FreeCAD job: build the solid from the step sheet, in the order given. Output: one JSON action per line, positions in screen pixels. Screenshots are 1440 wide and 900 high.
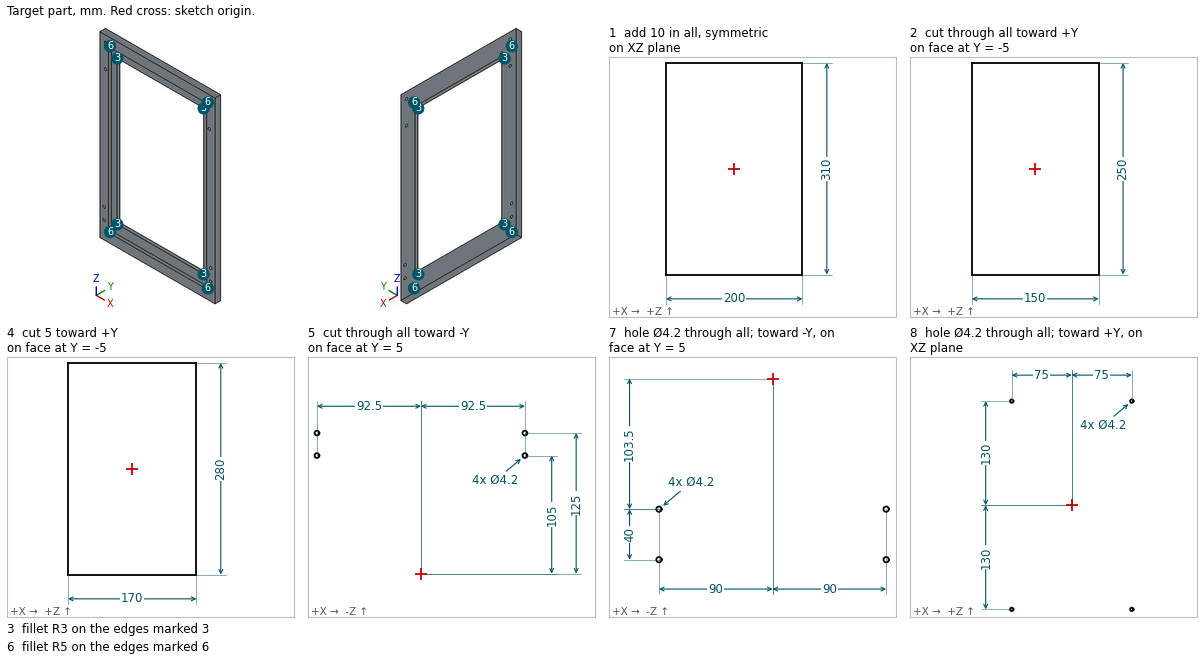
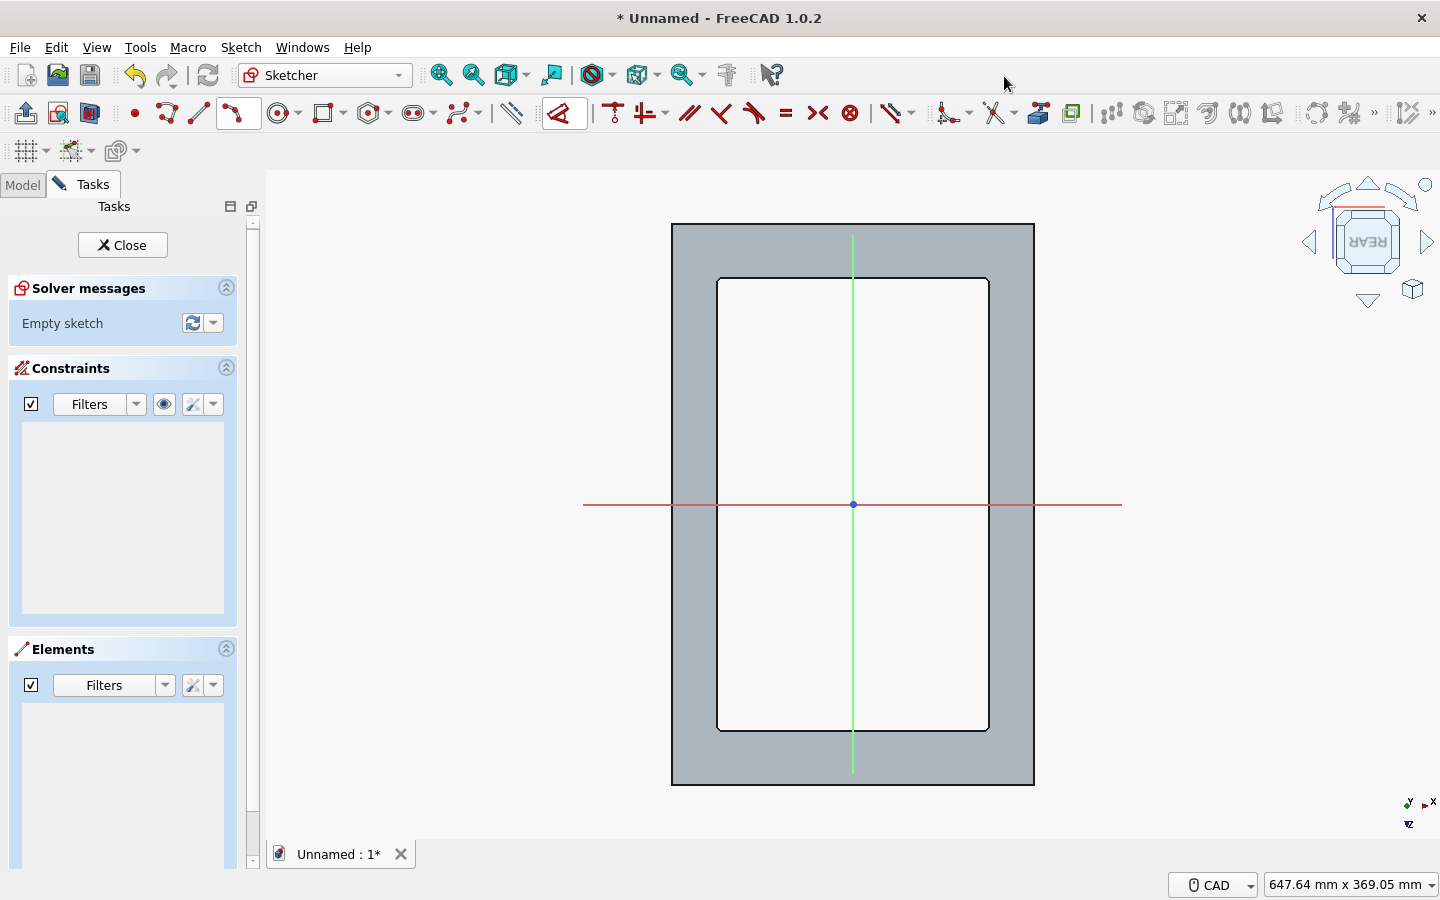
{"action": "scroll", "coordinate": [936, 249], "scroll_direction": "up", "scroll_amount": 3}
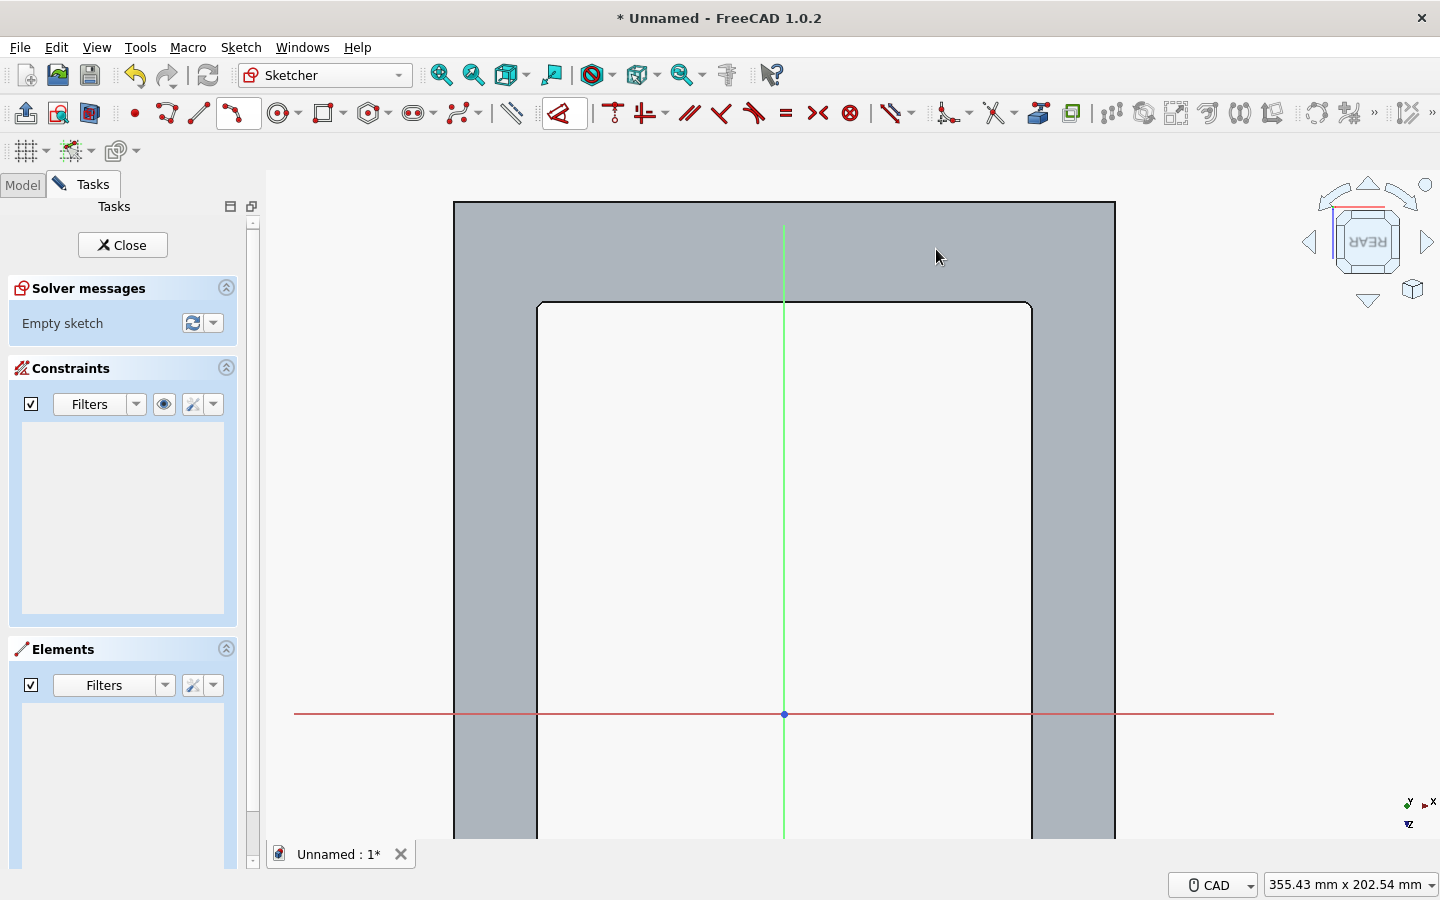
{"action": "key", "text": "g c"}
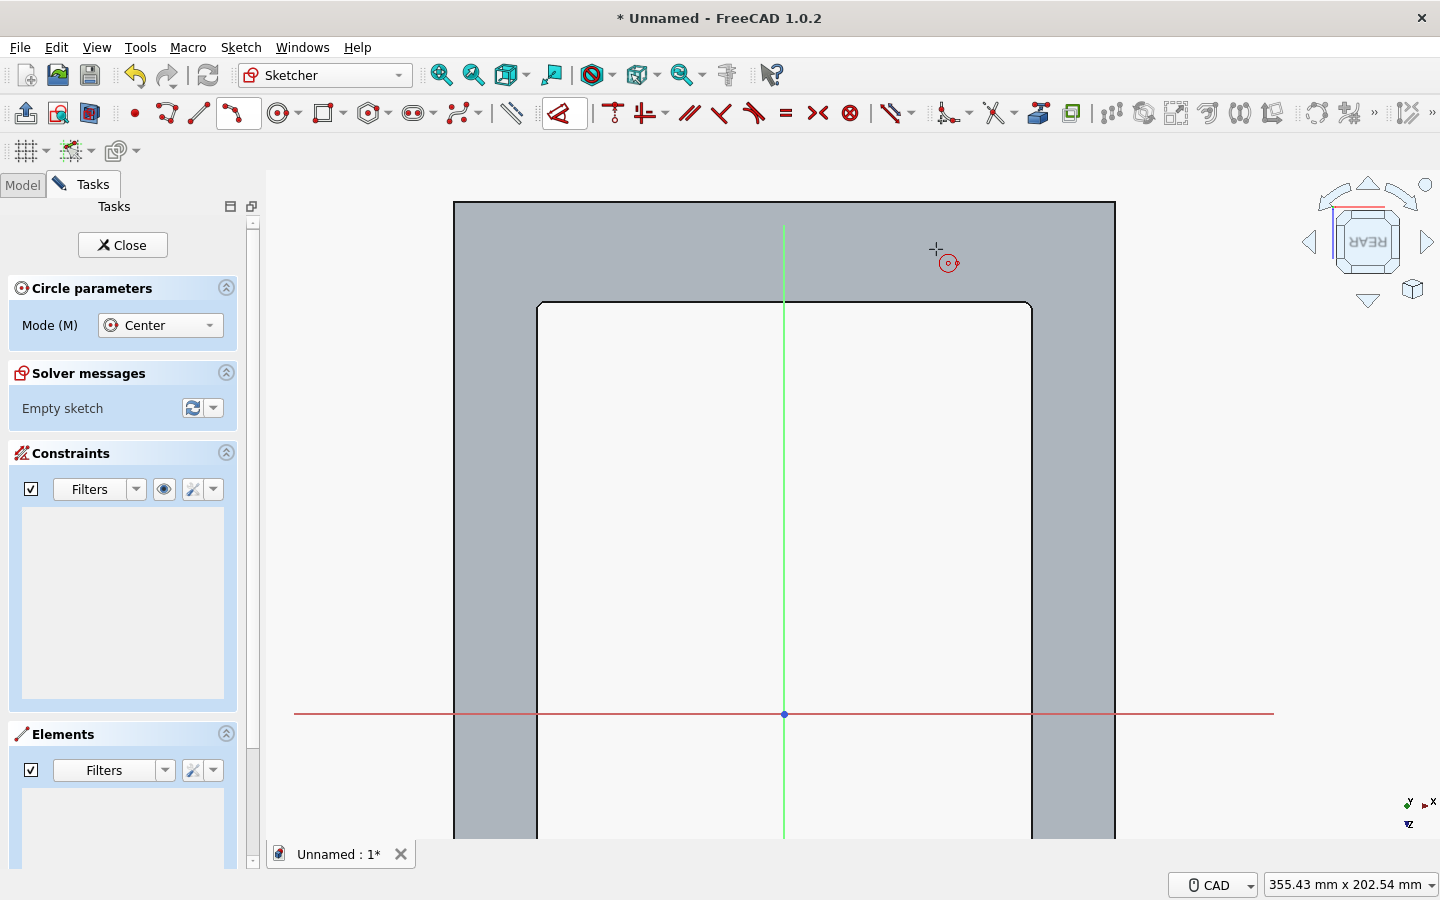
{"action": "scroll", "coordinate": [1090, 368], "scroll_direction": "up", "scroll_amount": 6}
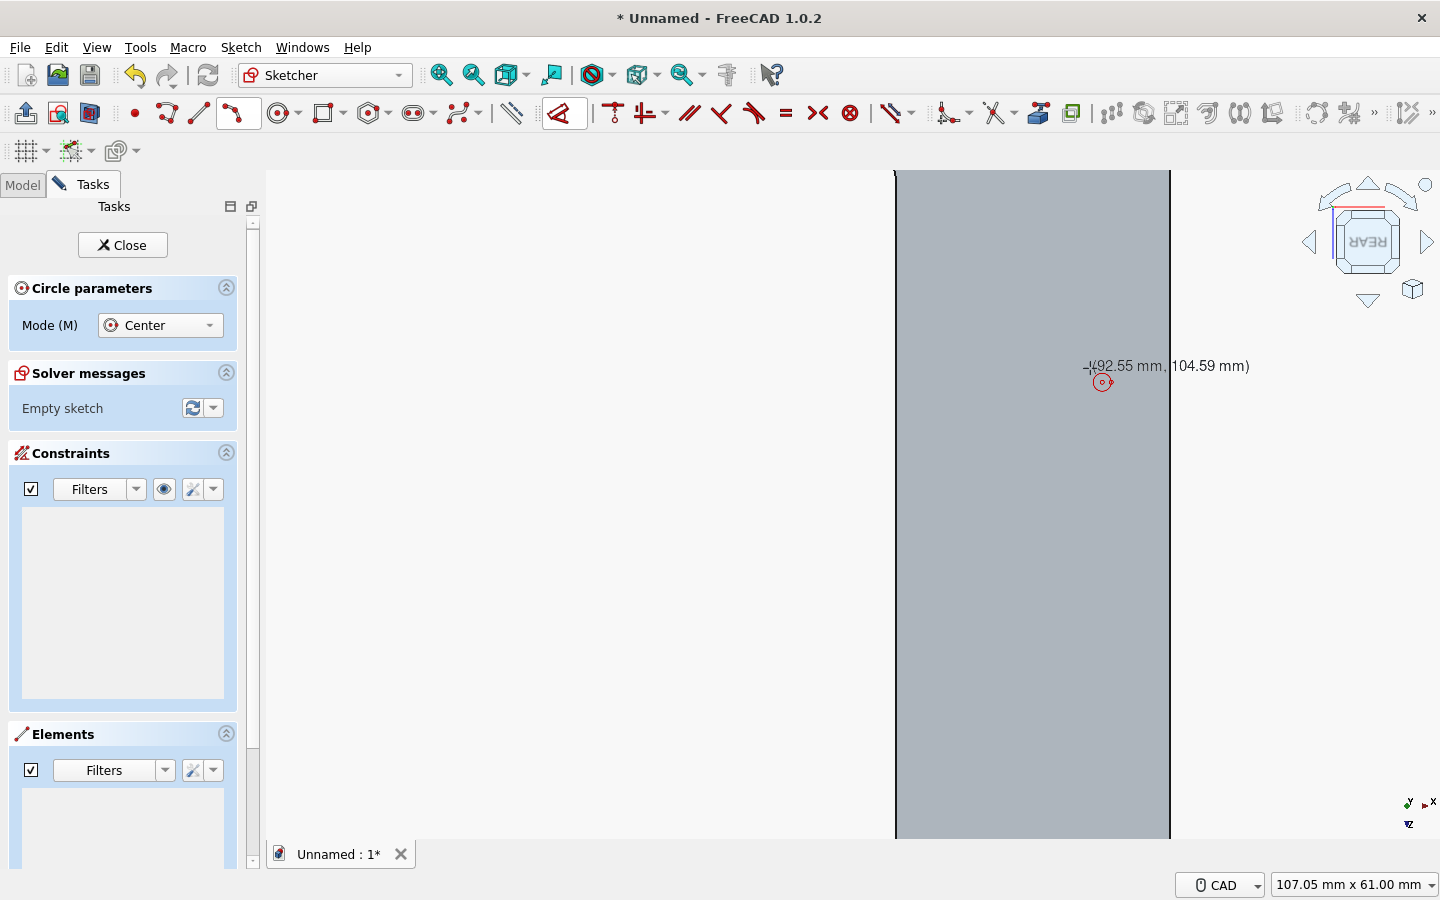
{"action": "left_click", "coordinate": [1088, 366]}
{"action": "left_click", "coordinate": [1104, 350]}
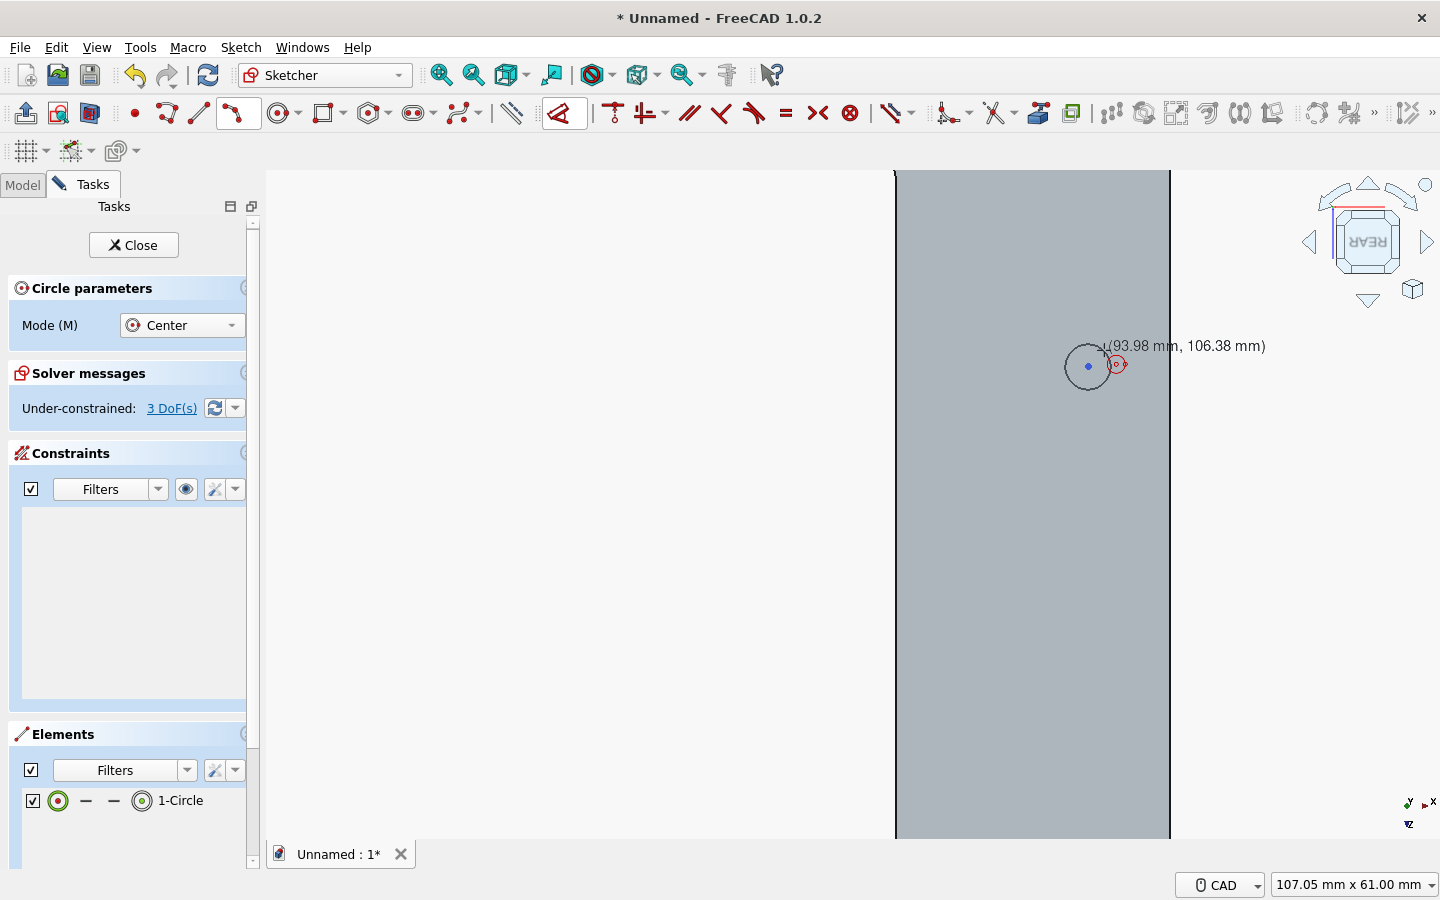
{"action": "scroll", "coordinate": [1091, 368], "scroll_direction": "down", "scroll_amount": 6}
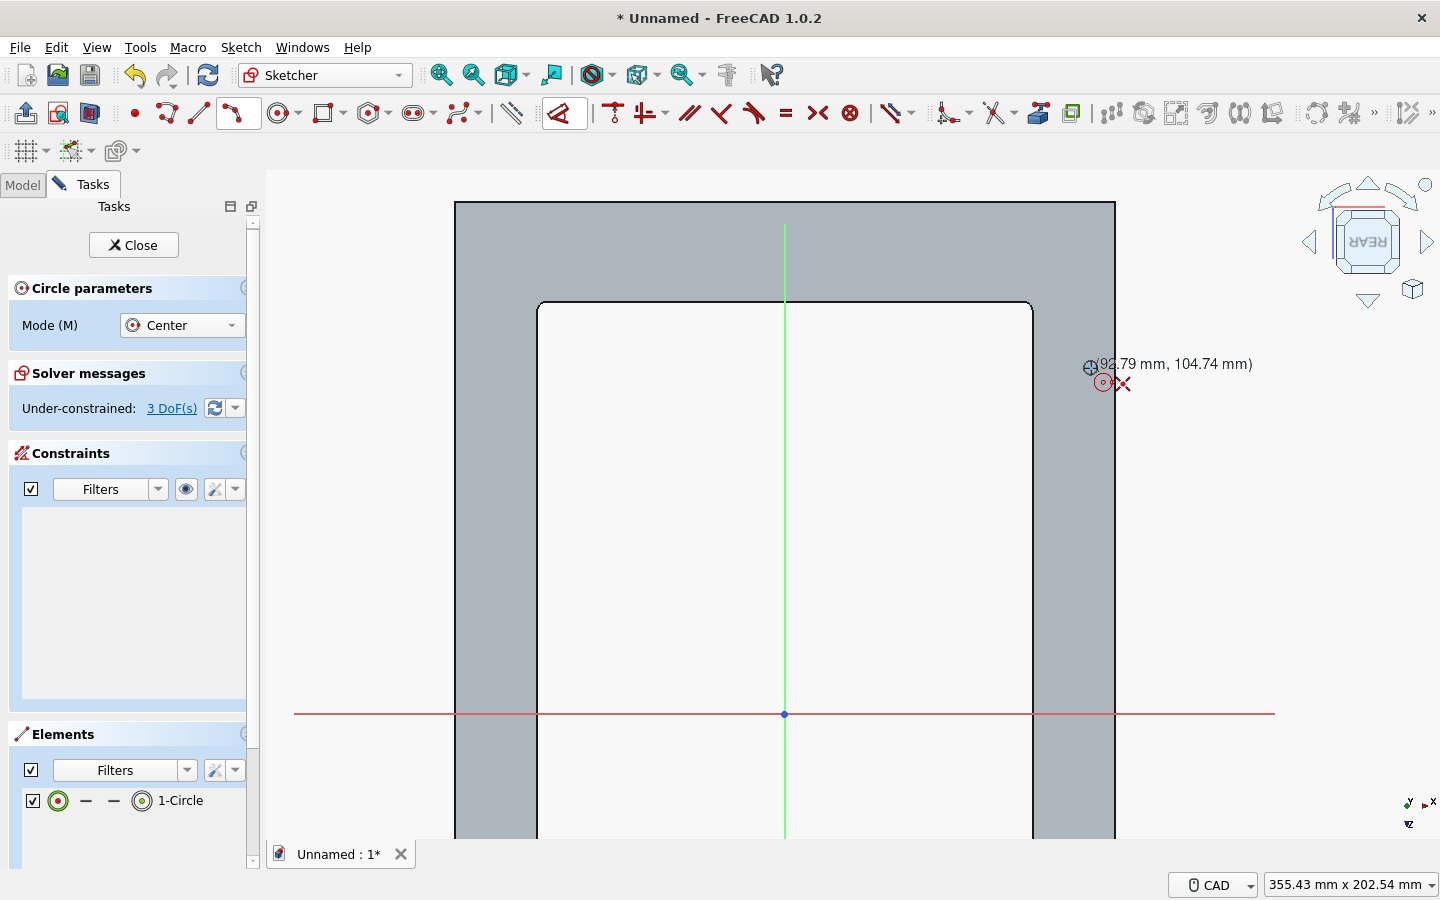
{"action": "scroll", "coordinate": [1091, 302], "scroll_direction": "up", "scroll_amount": 6}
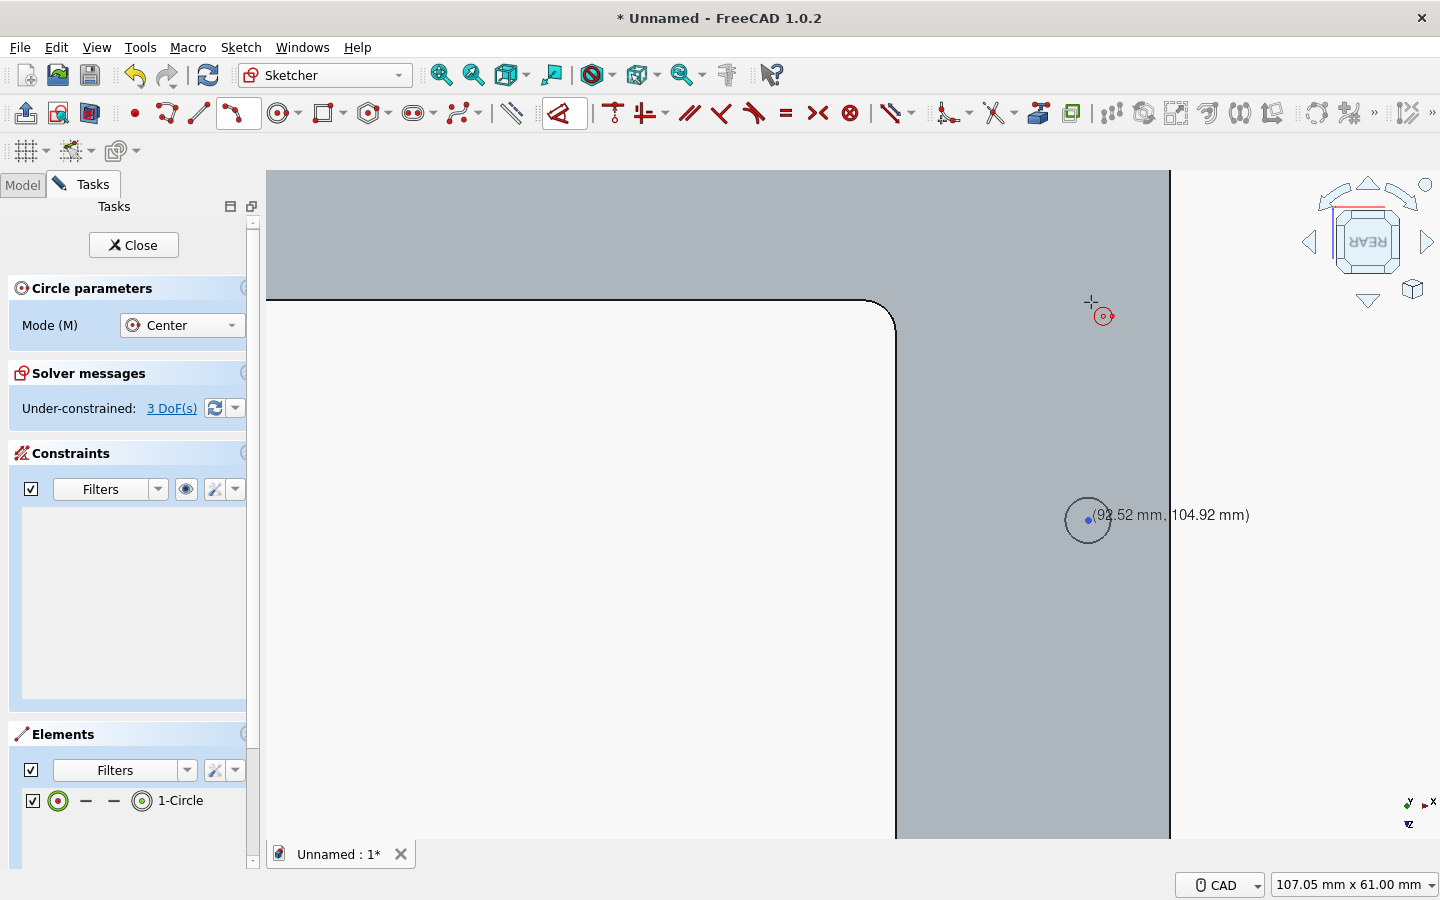
{"action": "left_click", "coordinate": [1088, 300]}
{"action": "left_click", "coordinate": [1104, 284]}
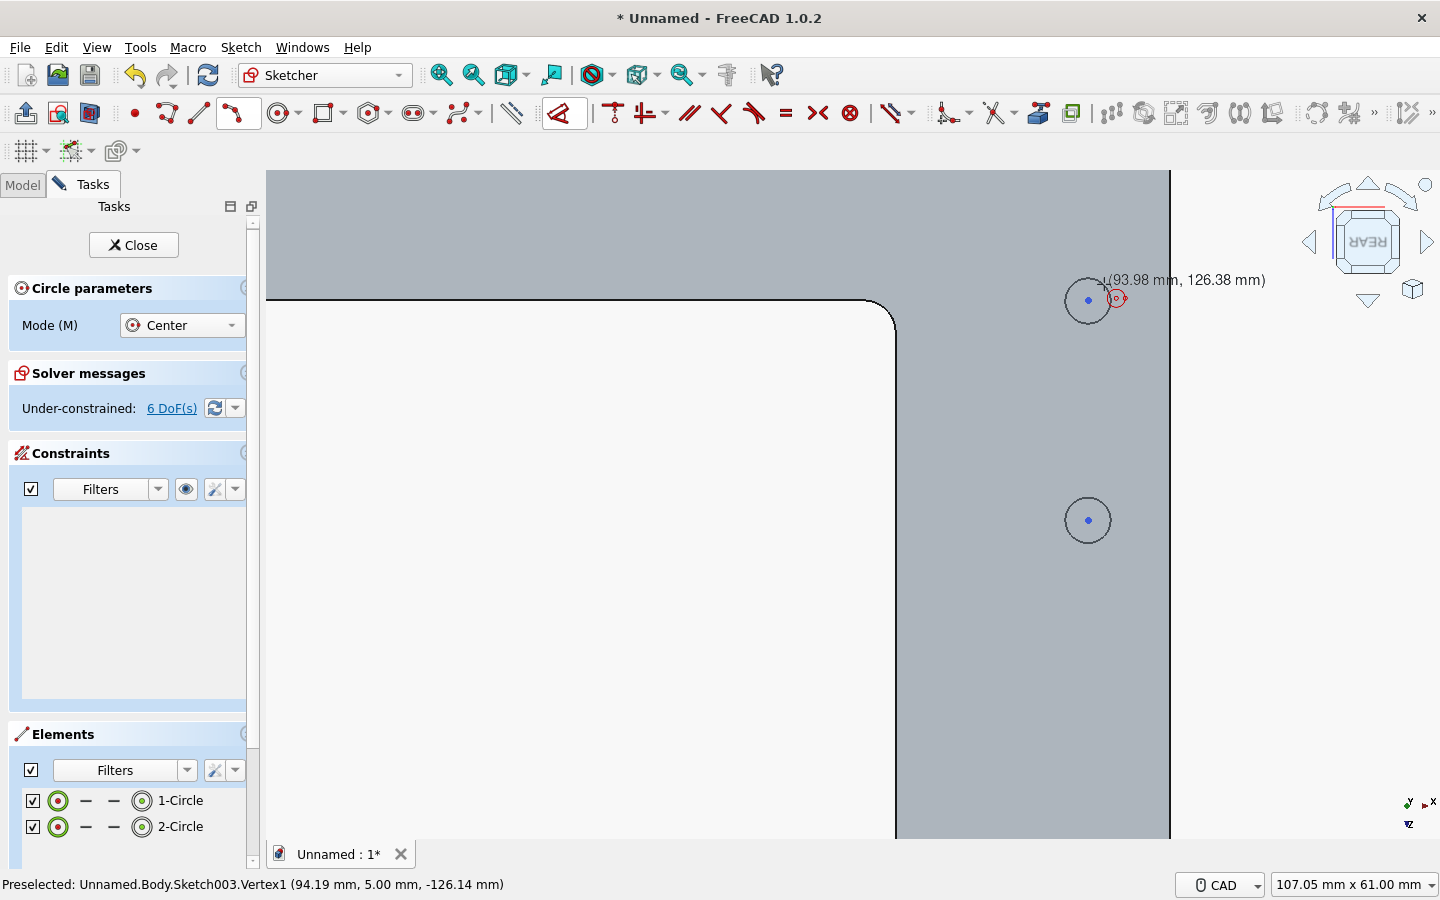
{"action": "scroll", "coordinate": [1091, 302], "scroll_direction": "down", "scroll_amount": 6}